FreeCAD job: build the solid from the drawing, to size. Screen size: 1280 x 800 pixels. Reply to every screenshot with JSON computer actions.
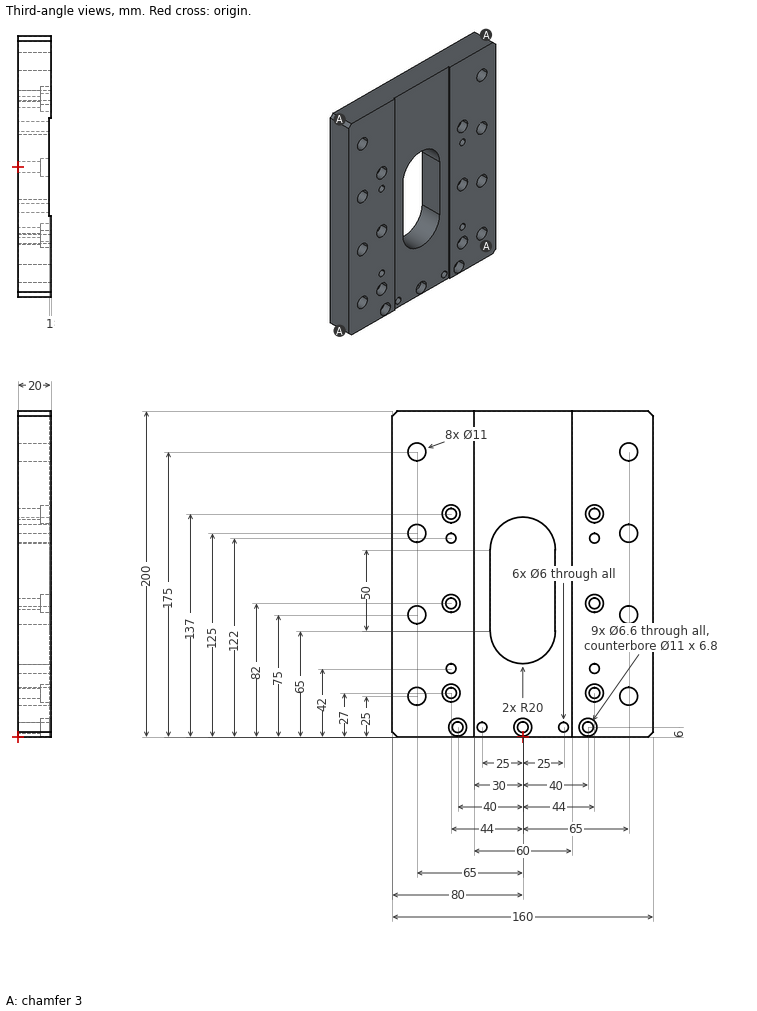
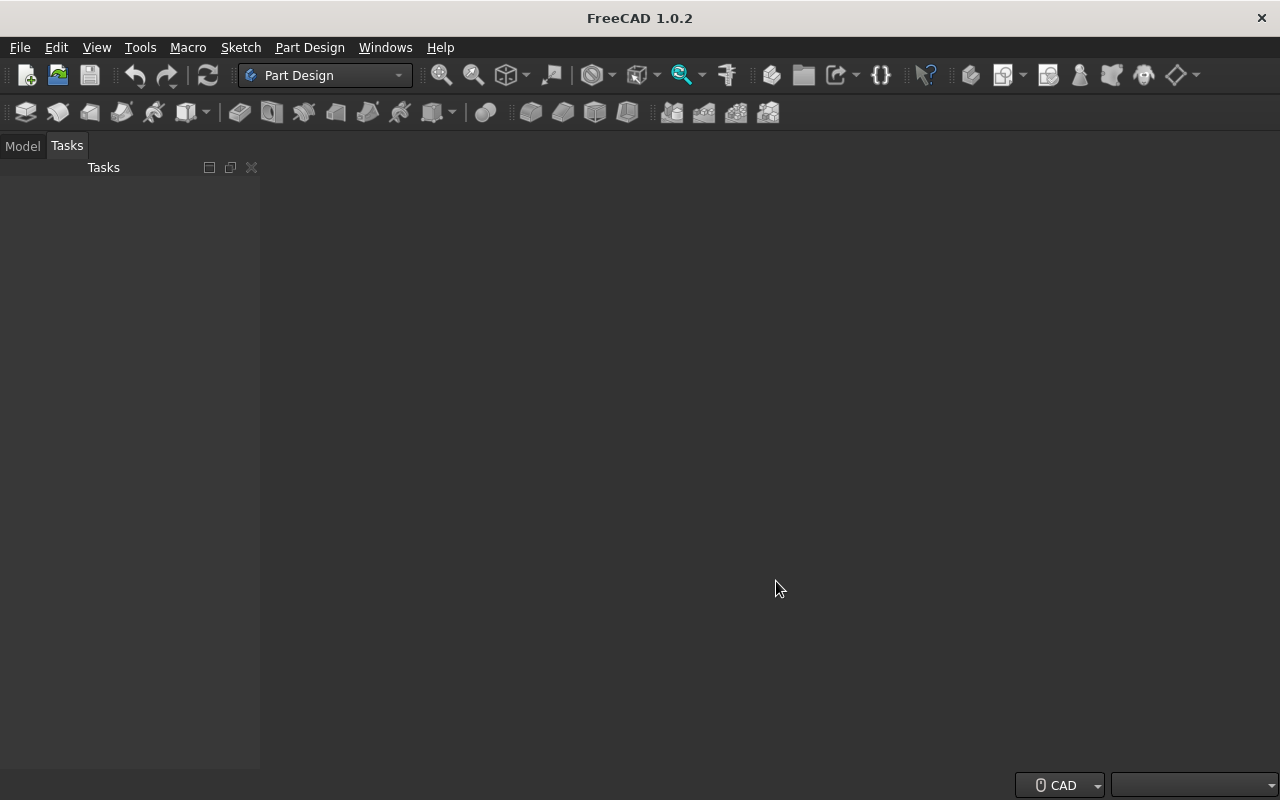
{"action": "key", "text": "ctrl+n"}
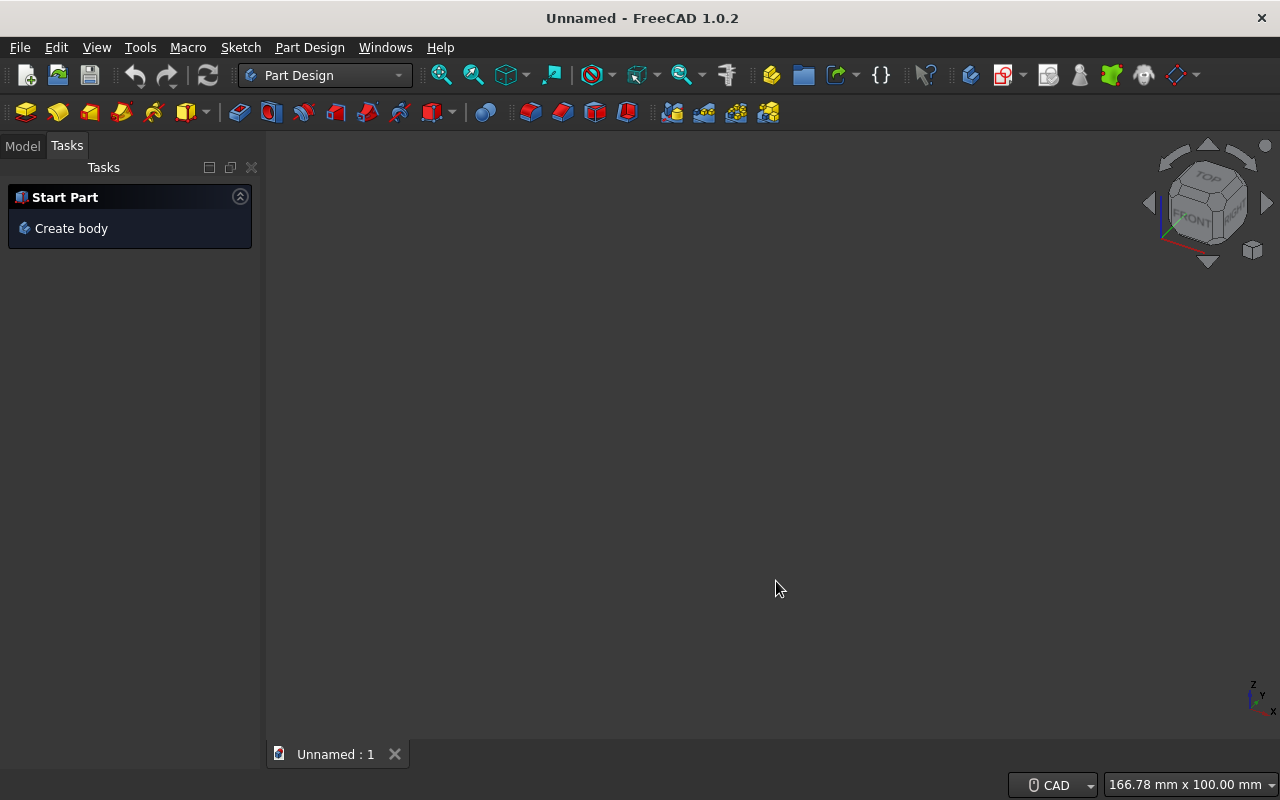
{"action": "left_click", "coordinate": [1004, 76]}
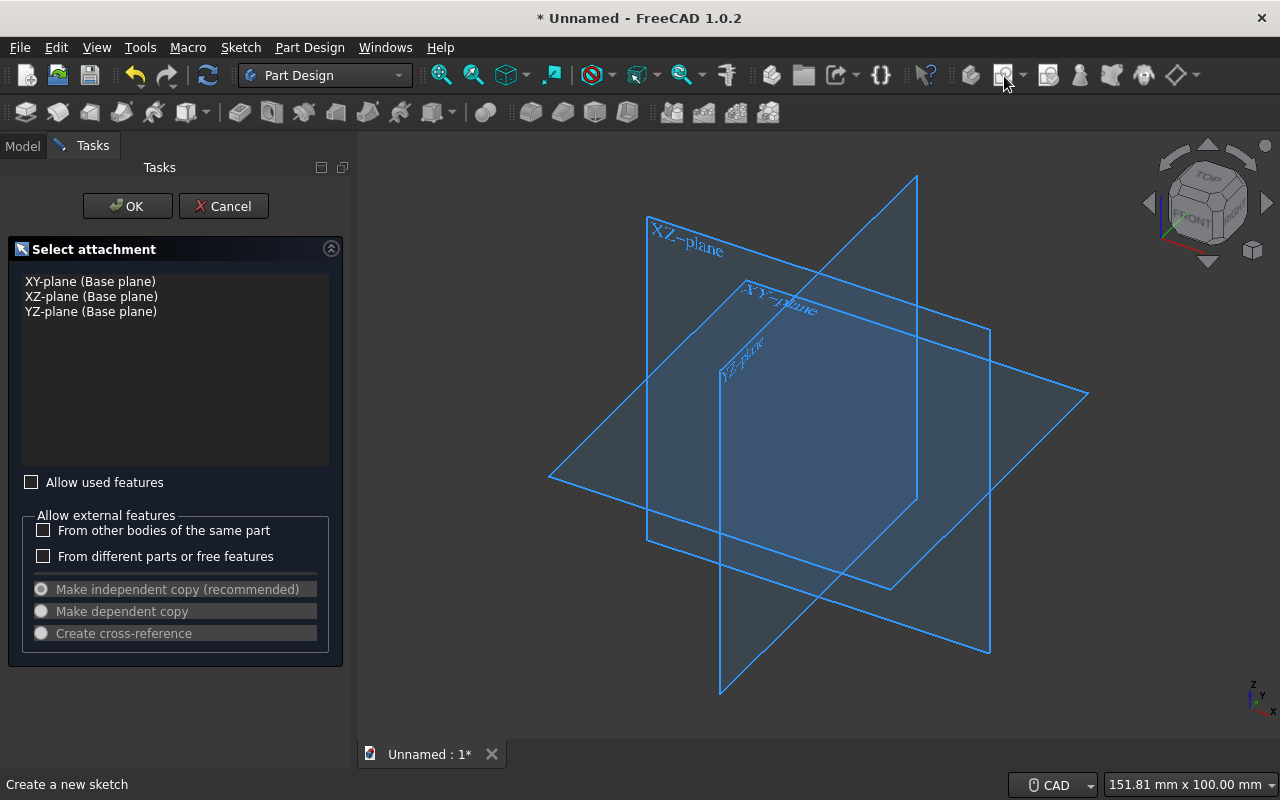
{"action": "left_click", "coordinate": [82, 312]}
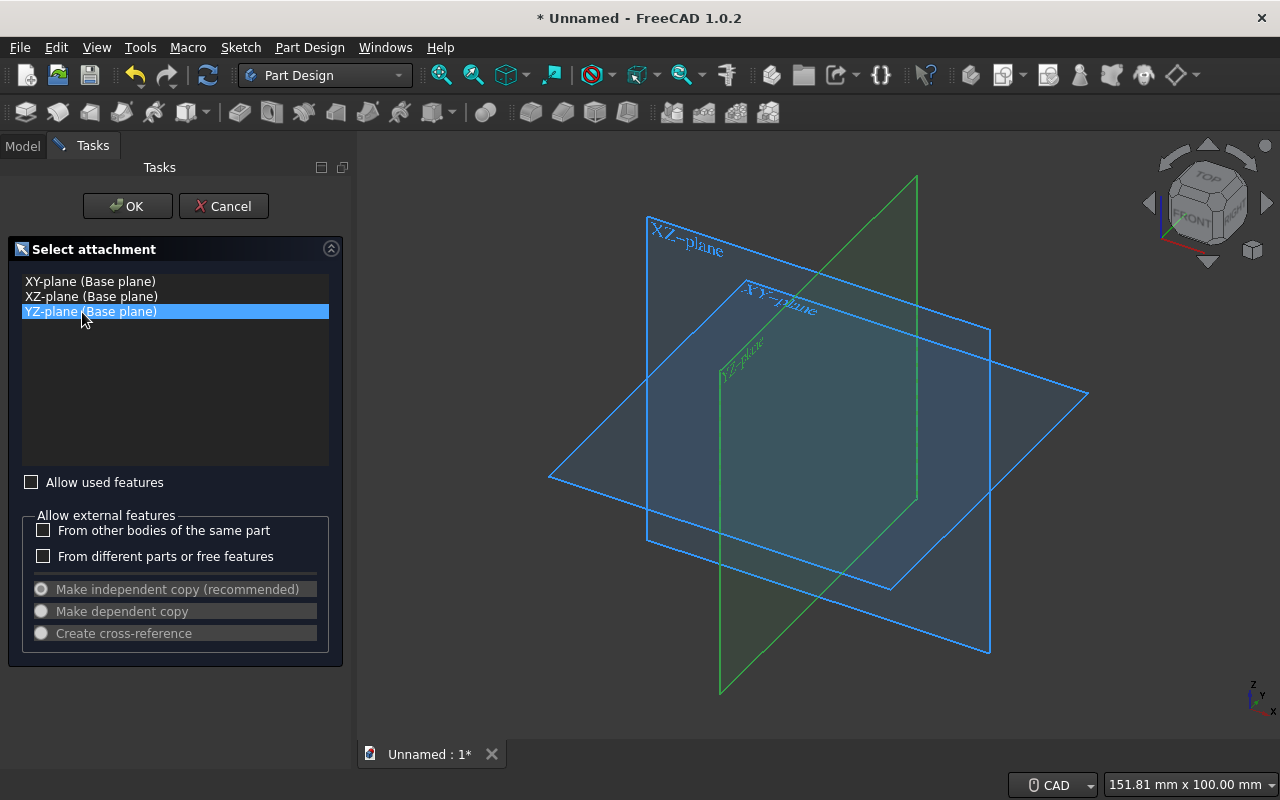
{"action": "left_click", "coordinate": [128, 206]}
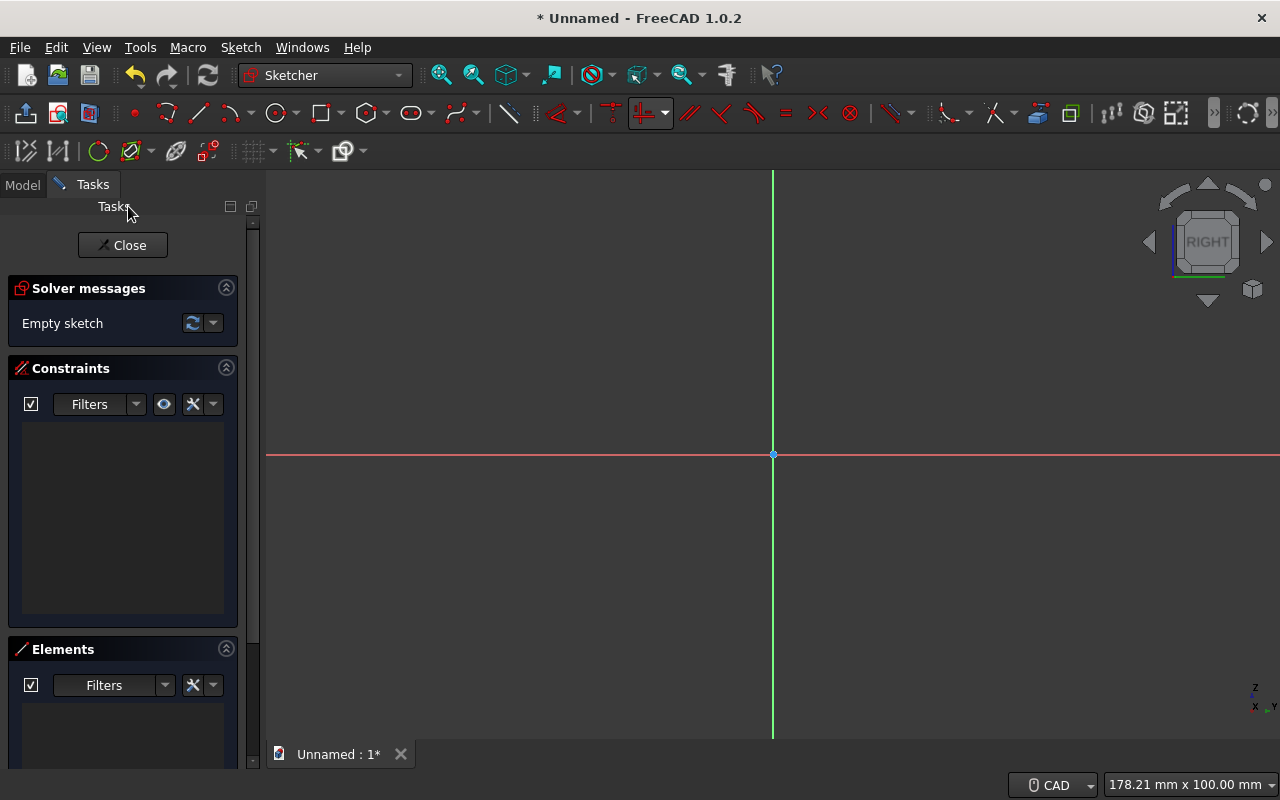
{"action": "scroll", "coordinate": [675, 700], "scroll_direction": "down", "scroll_amount": 6}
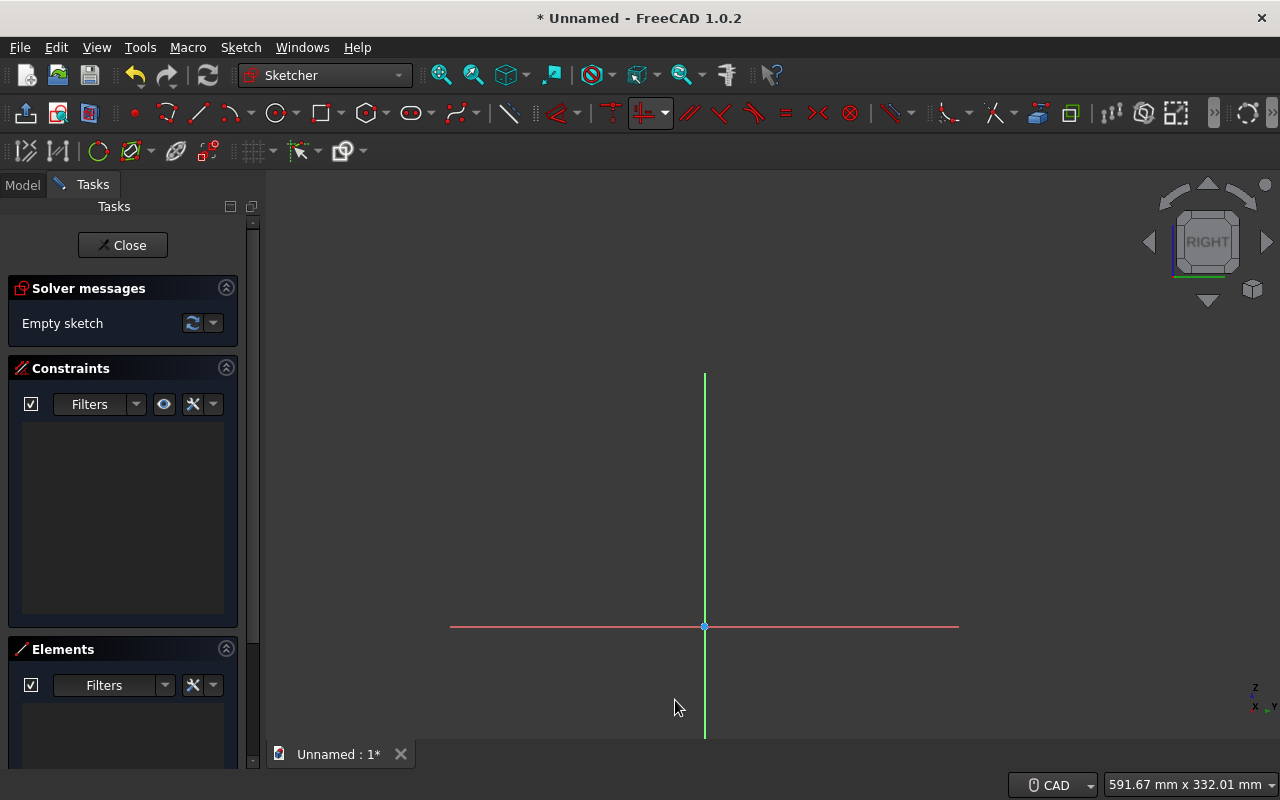
{"action": "key", "text": "g r"}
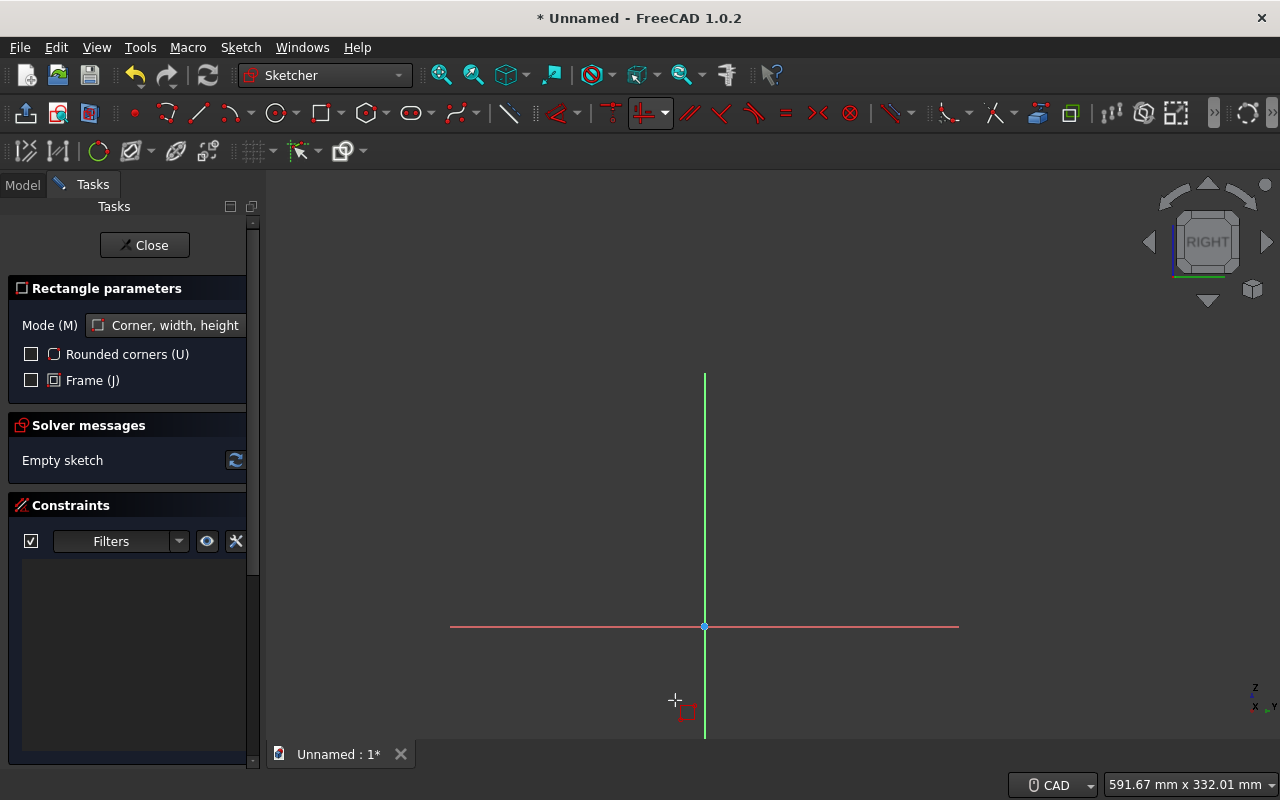
{"action": "left_click", "coordinate": [568, 284]}
{"action": "left_click", "coordinate": [842, 627]}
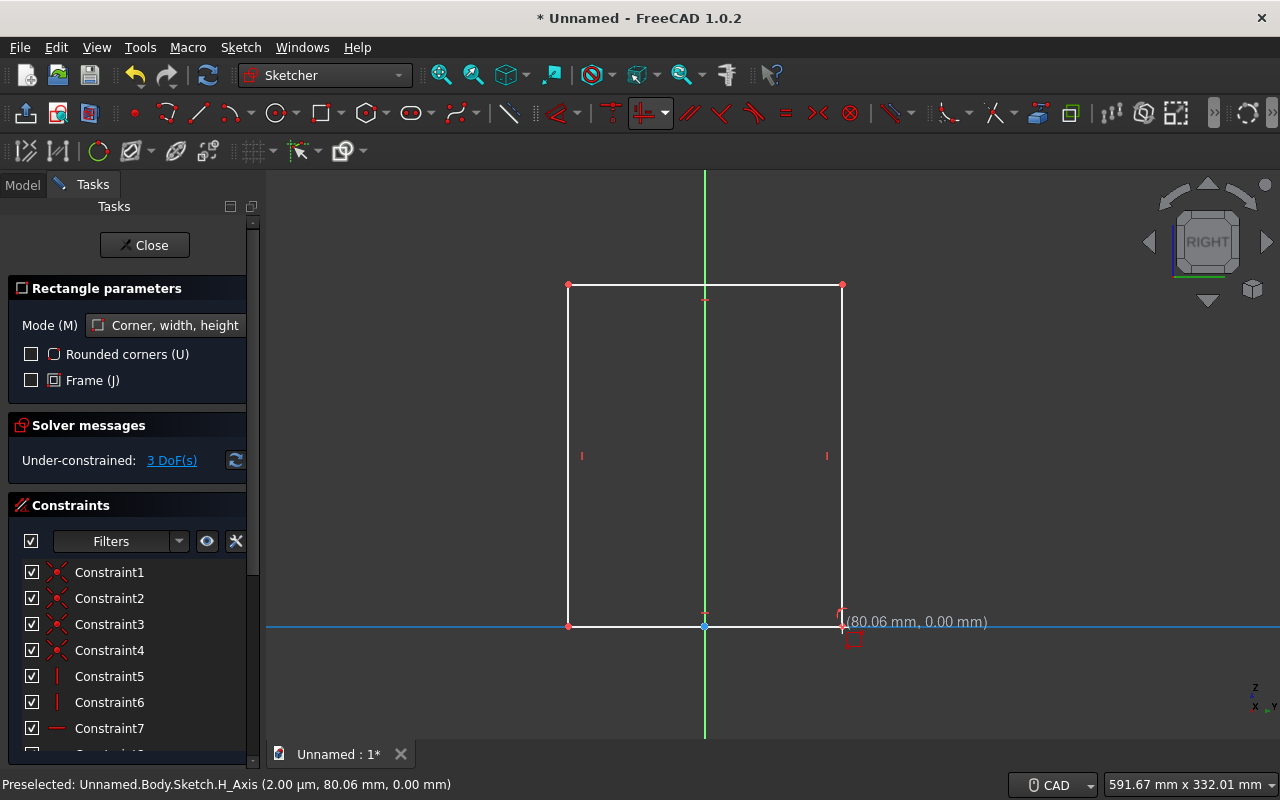
{"action": "key", "text": "g s"}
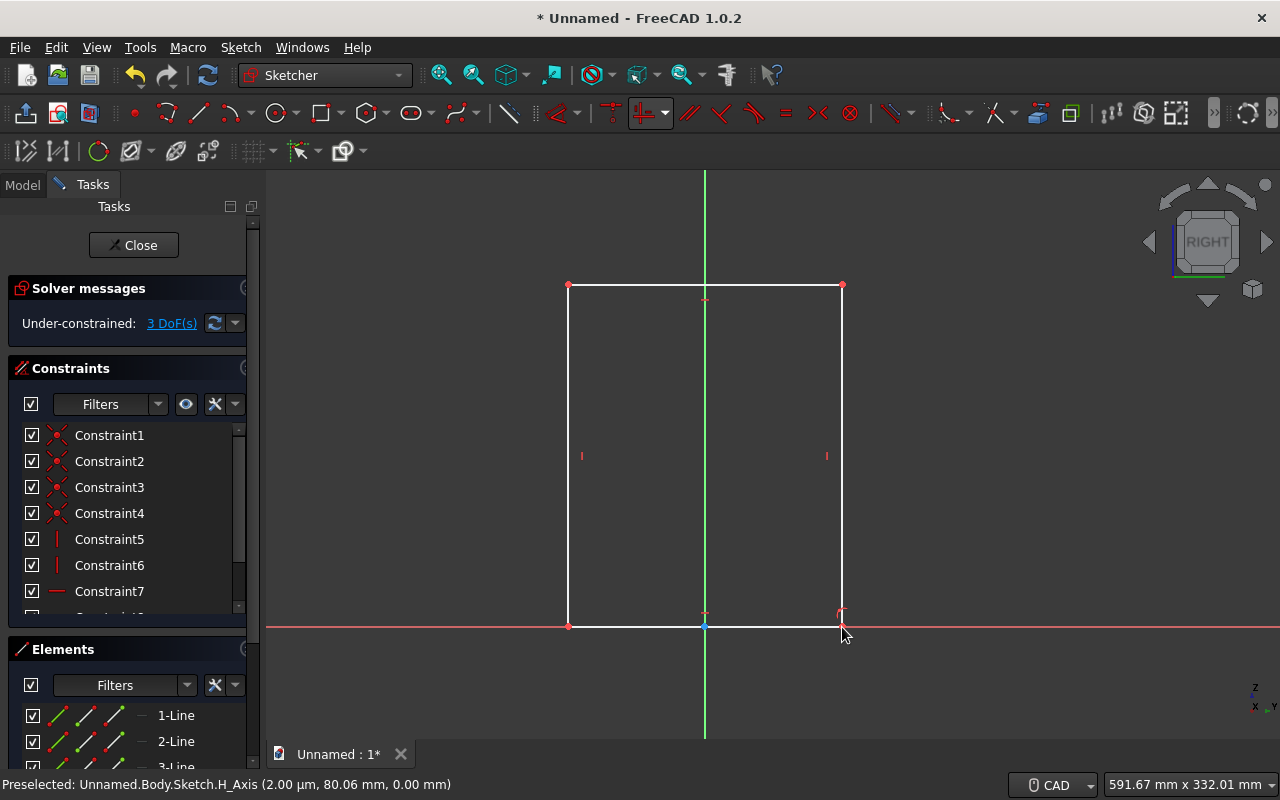
{"action": "left_click", "coordinate": [705, 515]}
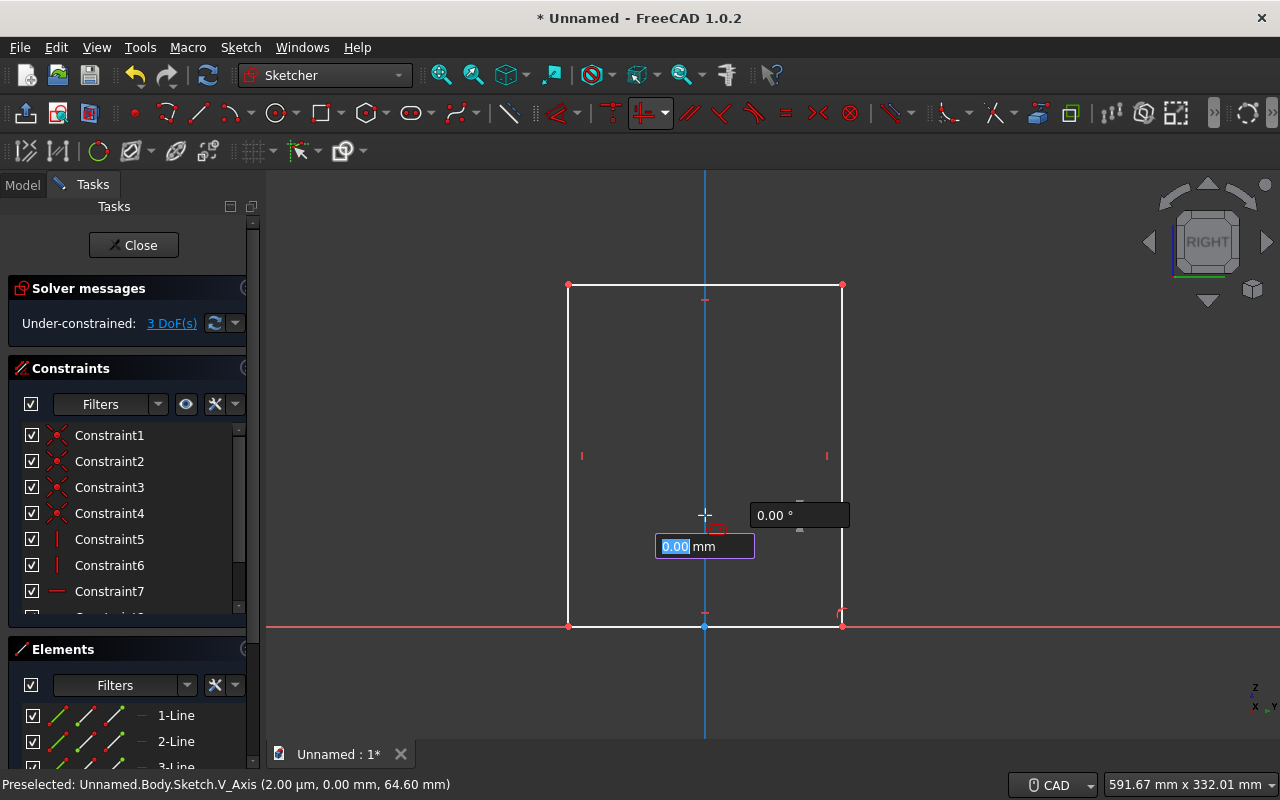
{"action": "left_click", "coordinate": [714, 430]}